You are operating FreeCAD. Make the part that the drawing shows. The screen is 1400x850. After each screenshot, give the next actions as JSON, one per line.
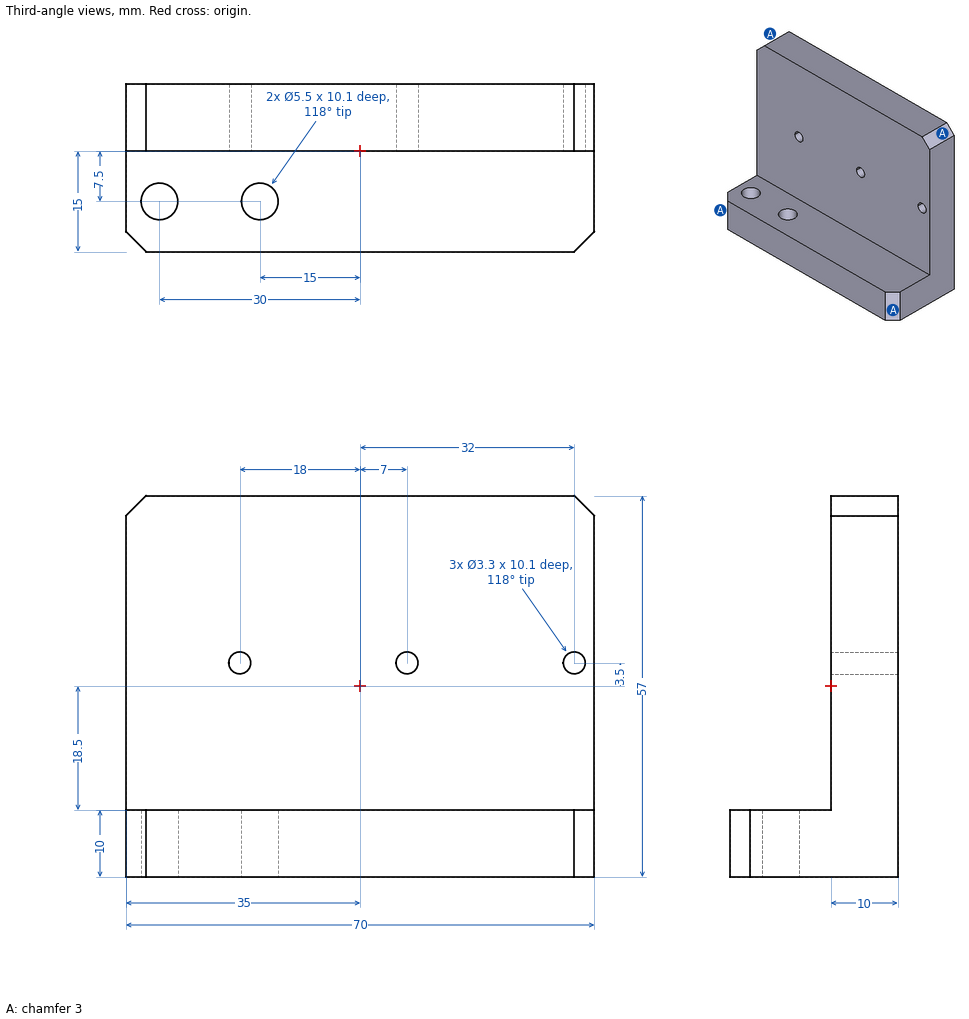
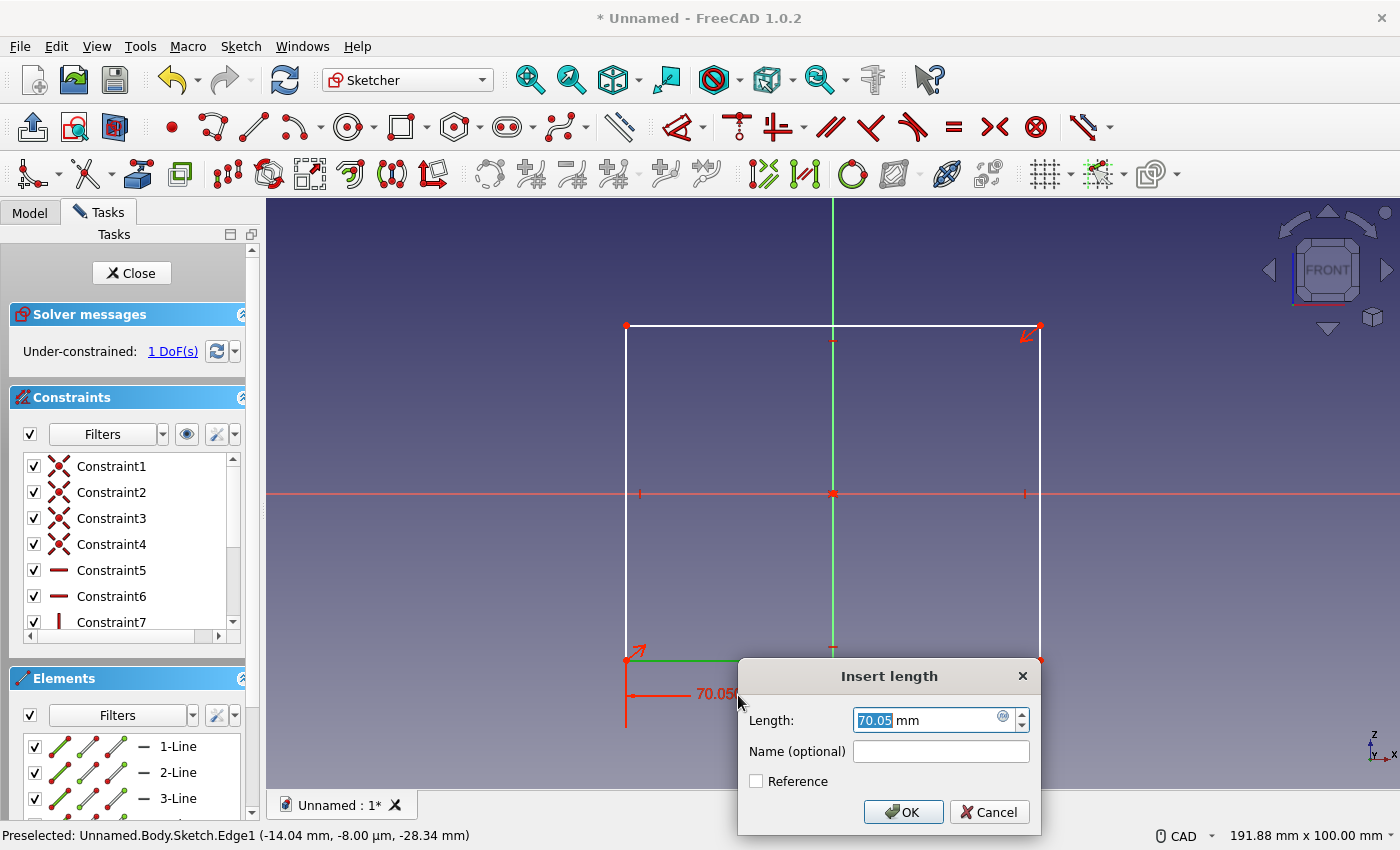
{"action": "type", "text": "70"}
{"action": "key", "text": "Return"}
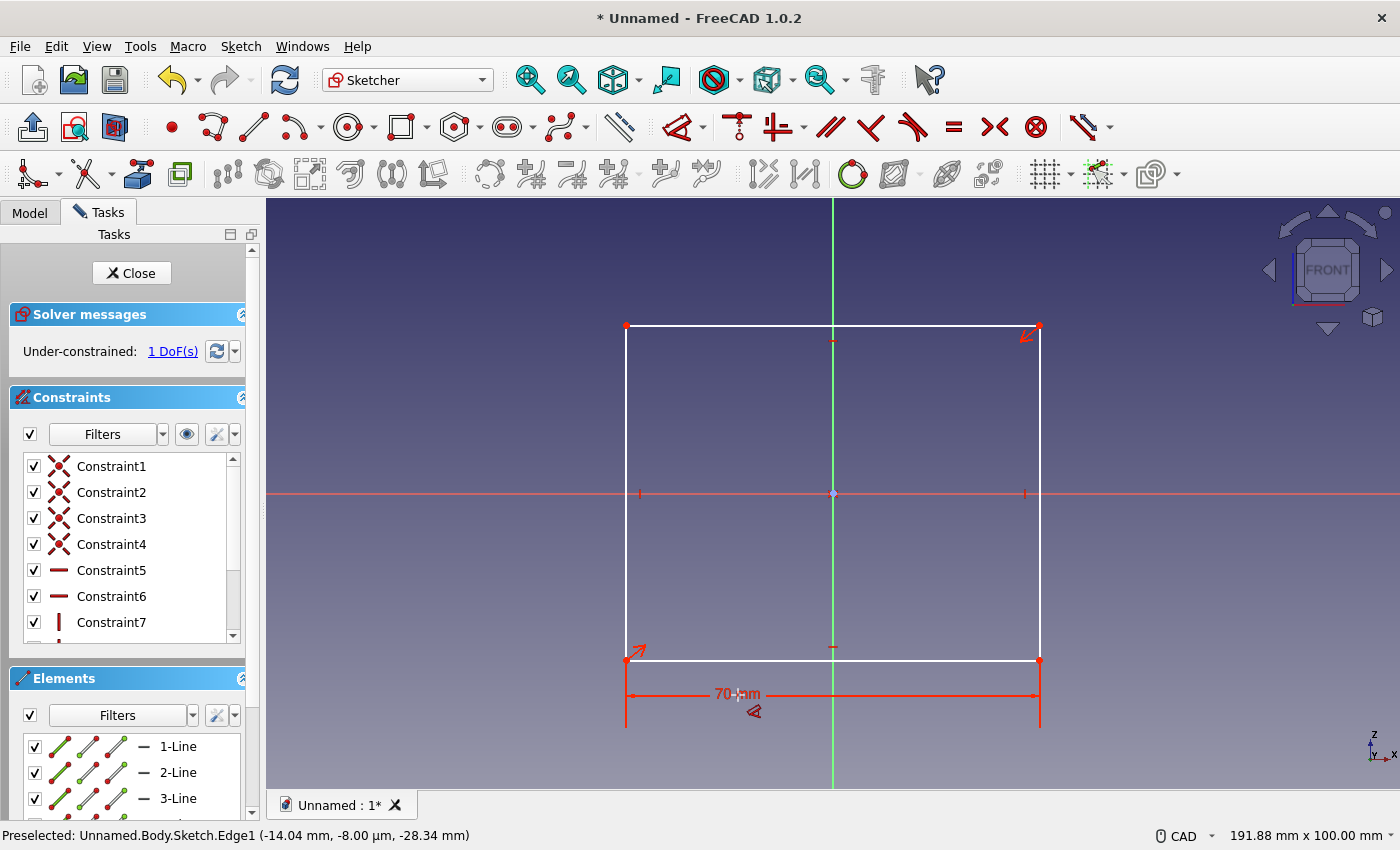
{"action": "left_click", "coordinate": [1040, 561]}
{"action": "left_click", "coordinate": [1074, 416]}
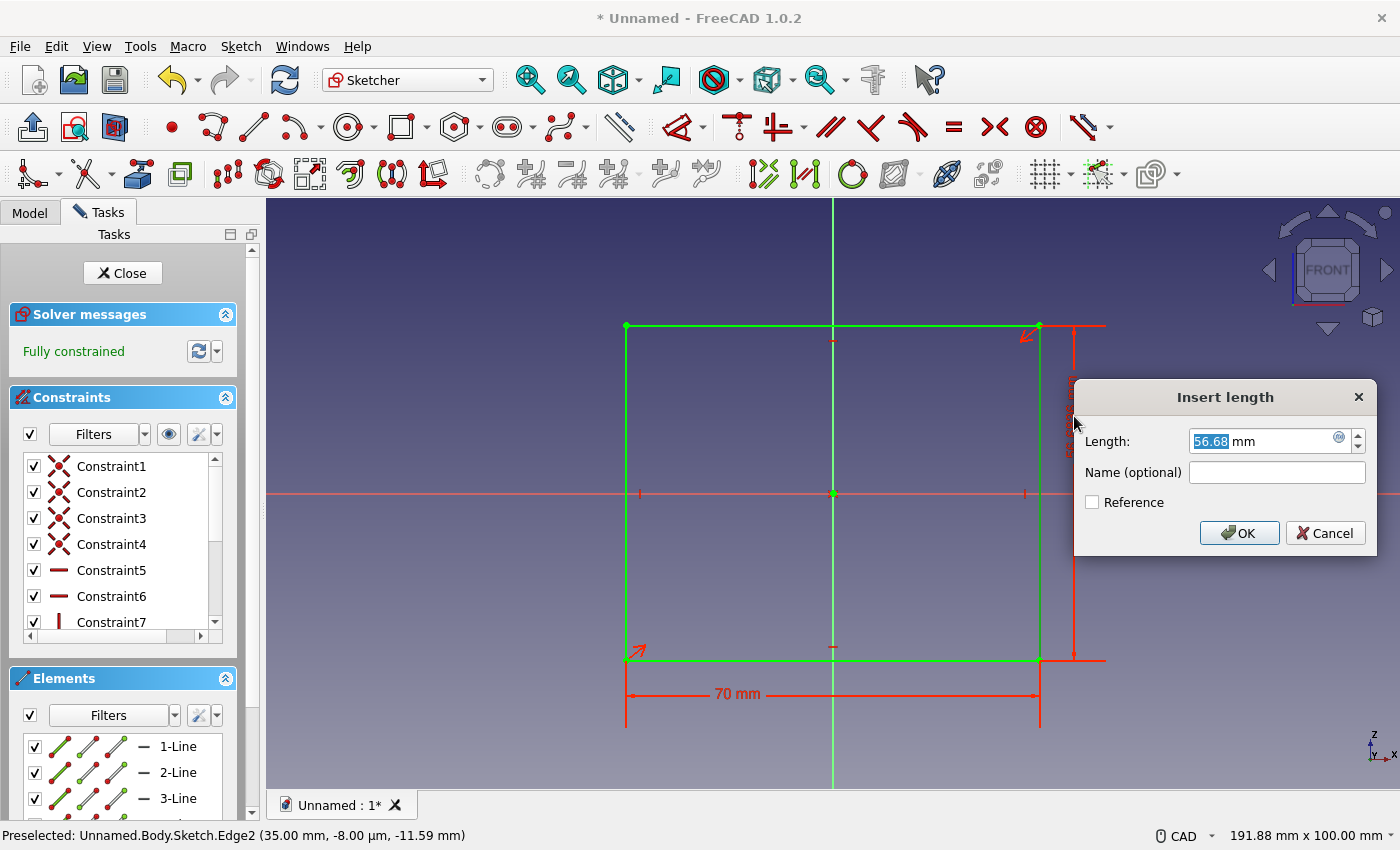
{"action": "type", "text": "57"}
{"action": "key", "text": "Return"}
{"action": "key", "text": "Escape"}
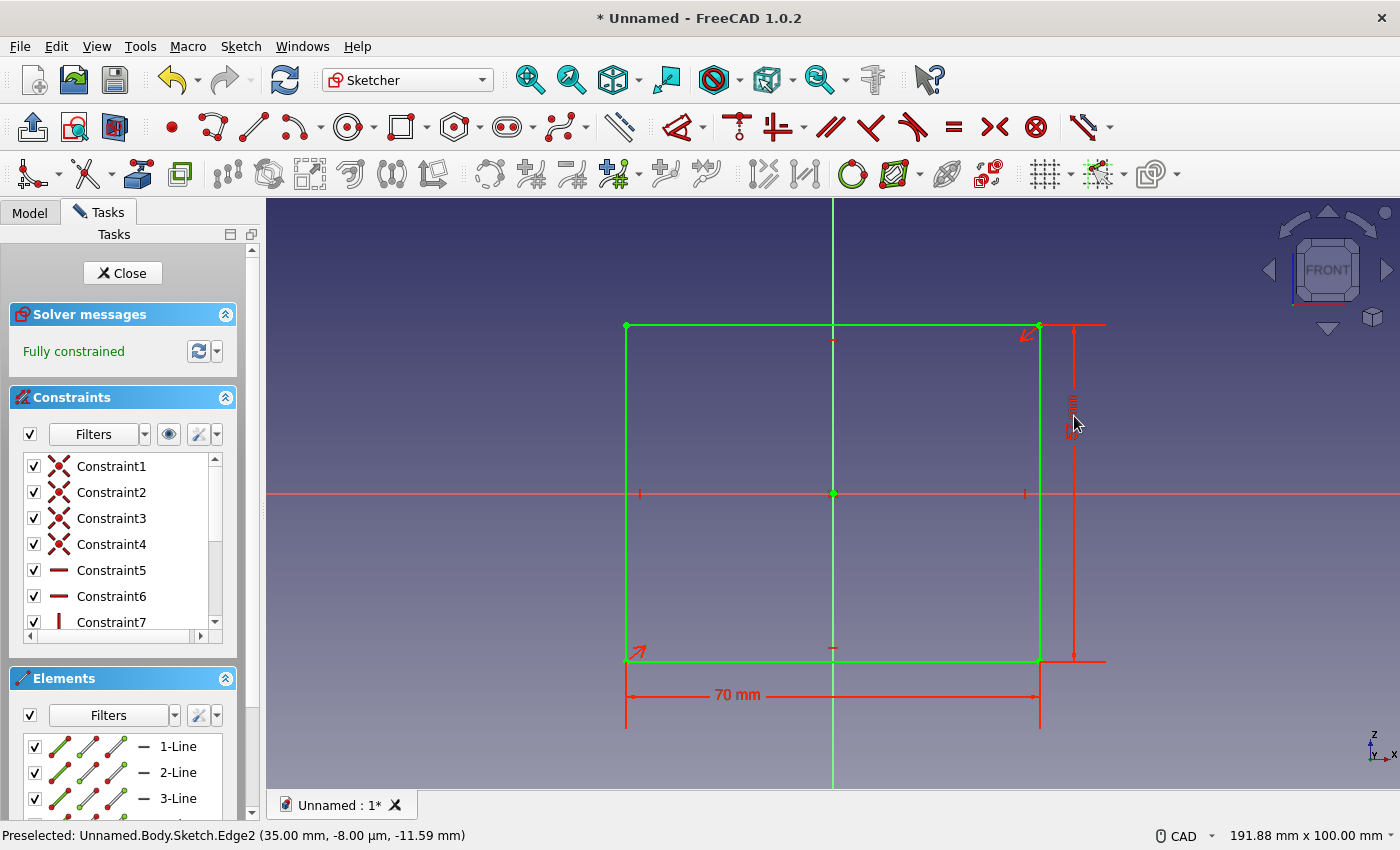
{"action": "left_click", "coordinate": [123, 273]}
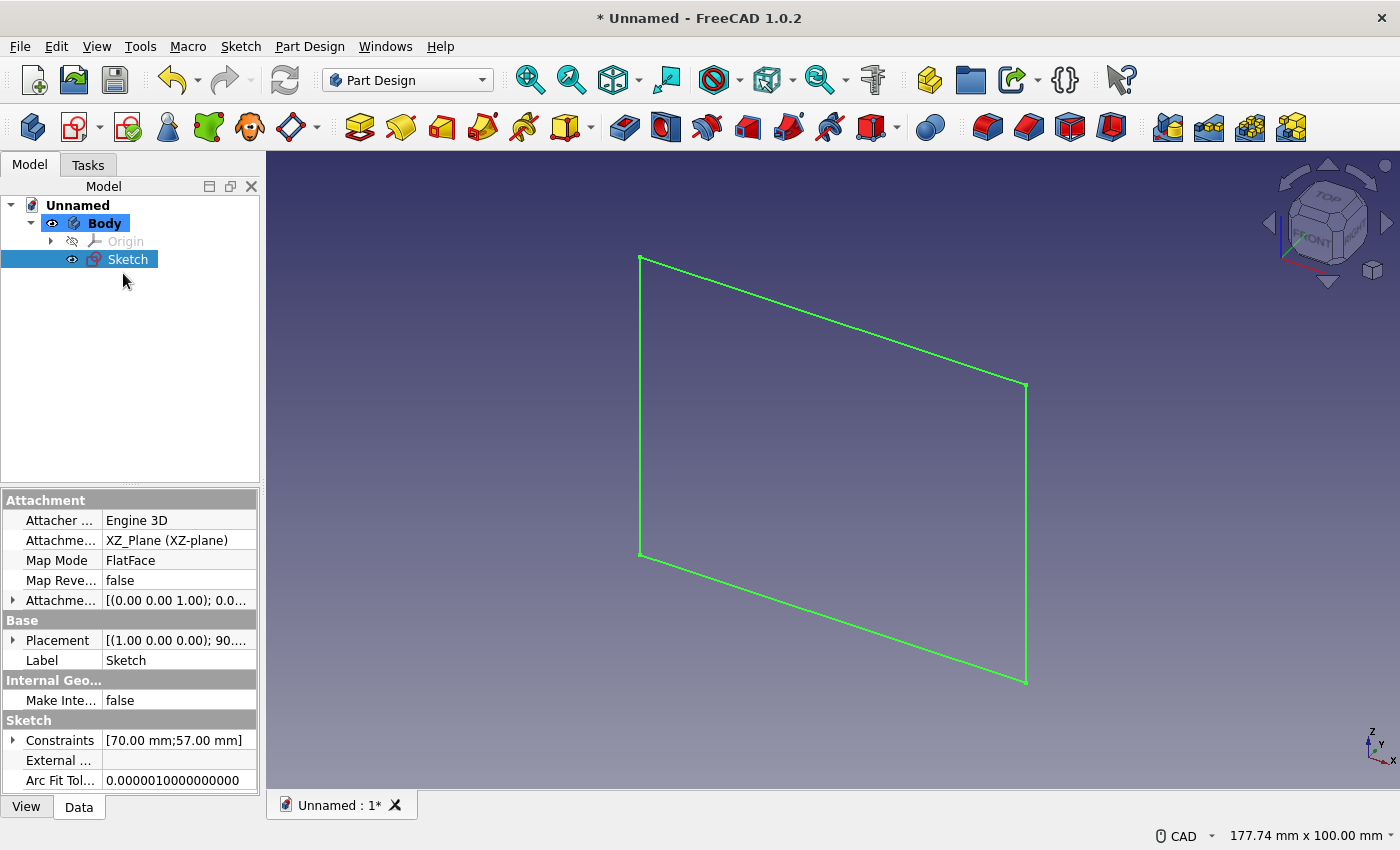
{"action": "left_click", "coordinate": [360, 128]}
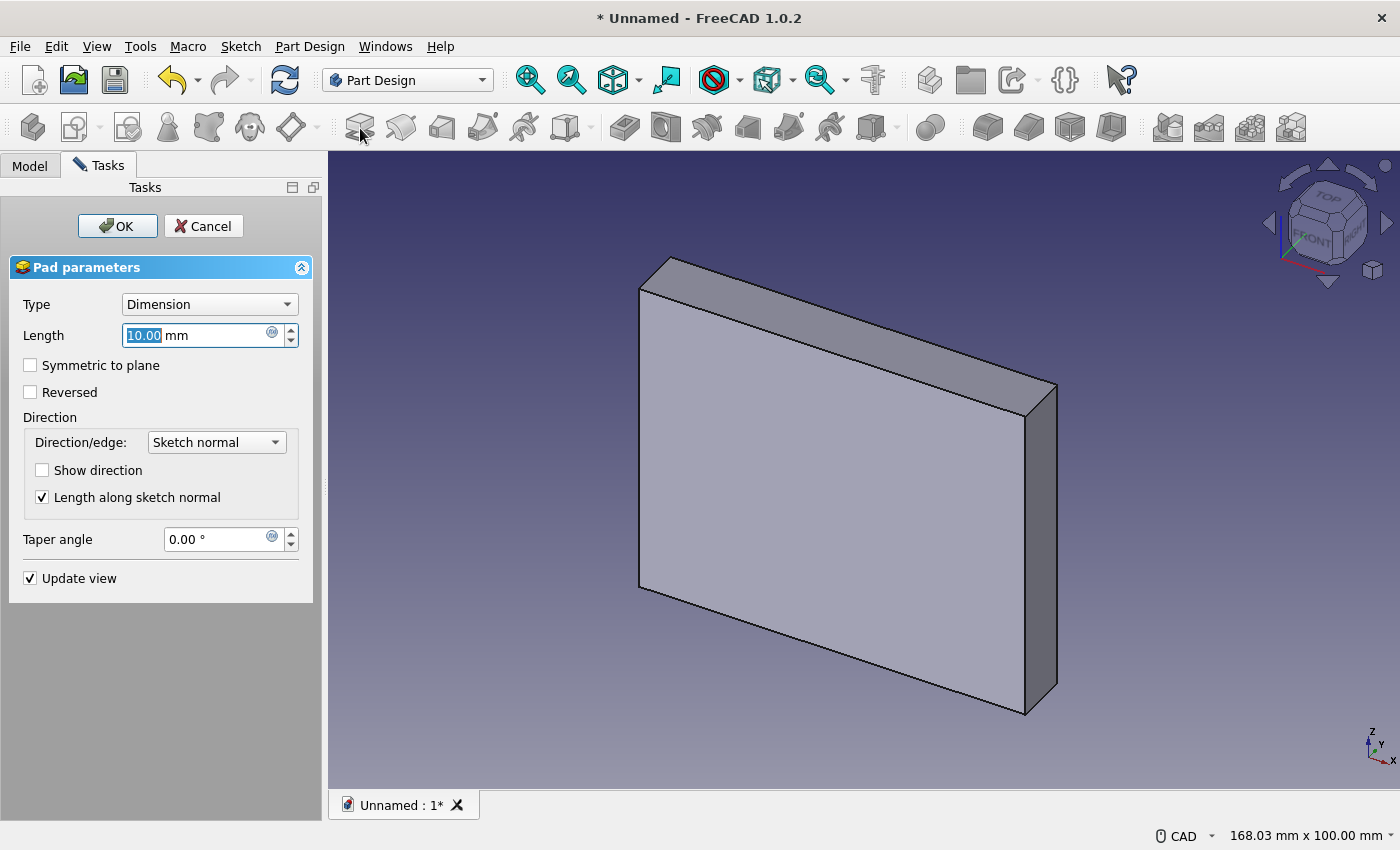
{"action": "type", "text": "10"}
{"action": "key", "text": "Tab"}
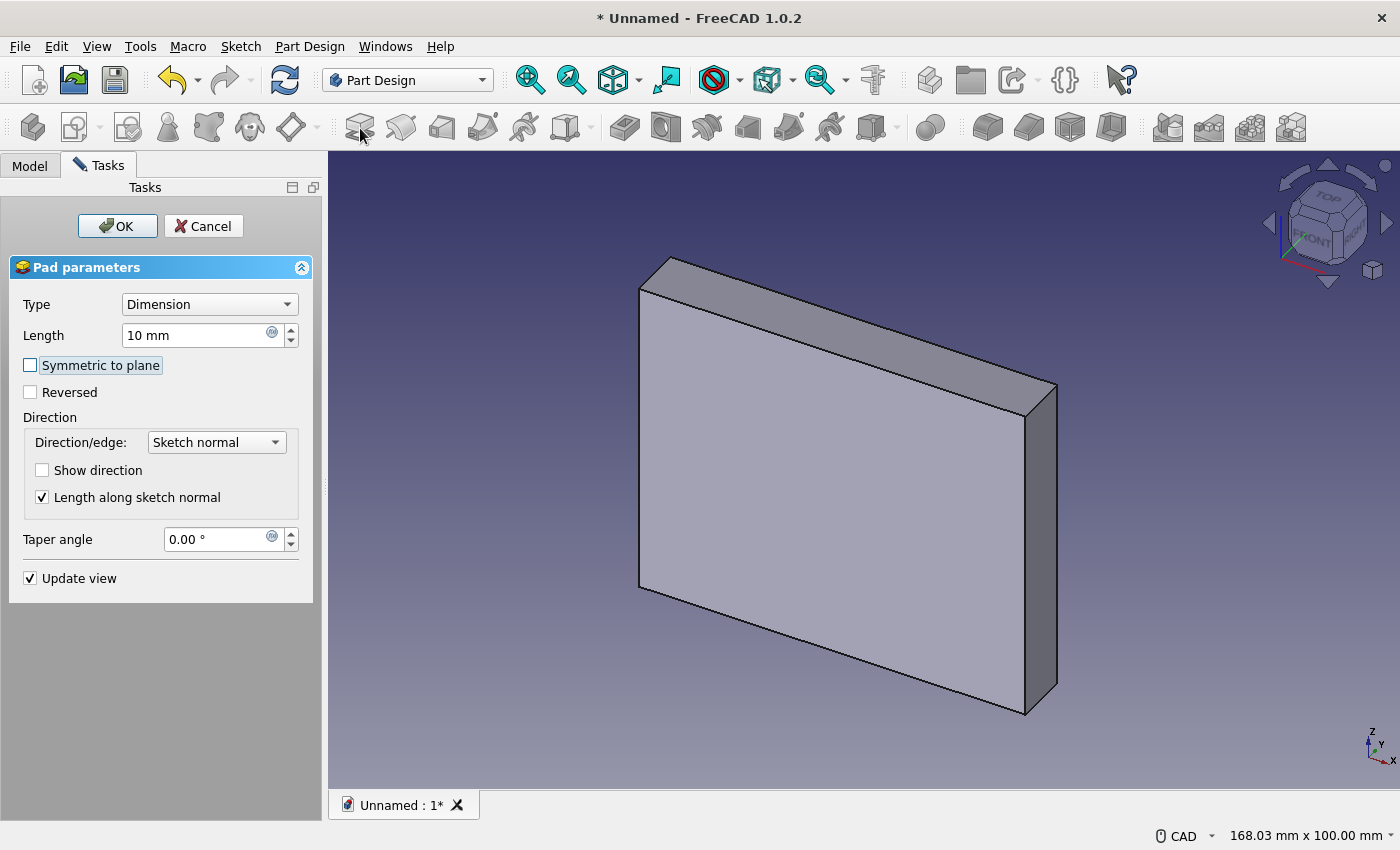
{"action": "left_click", "coordinate": [31, 392]}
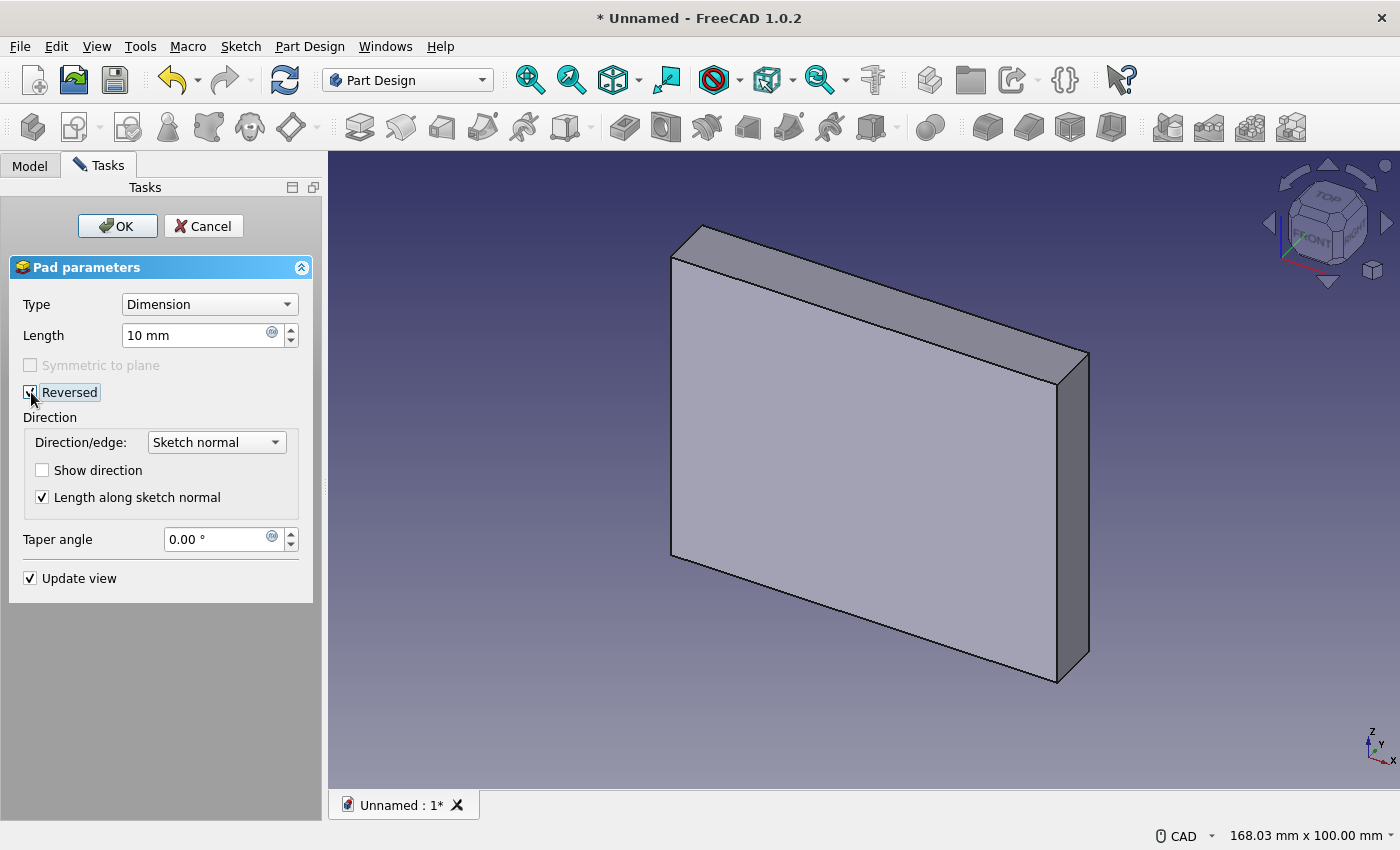
{"action": "left_click", "coordinate": [118, 226]}